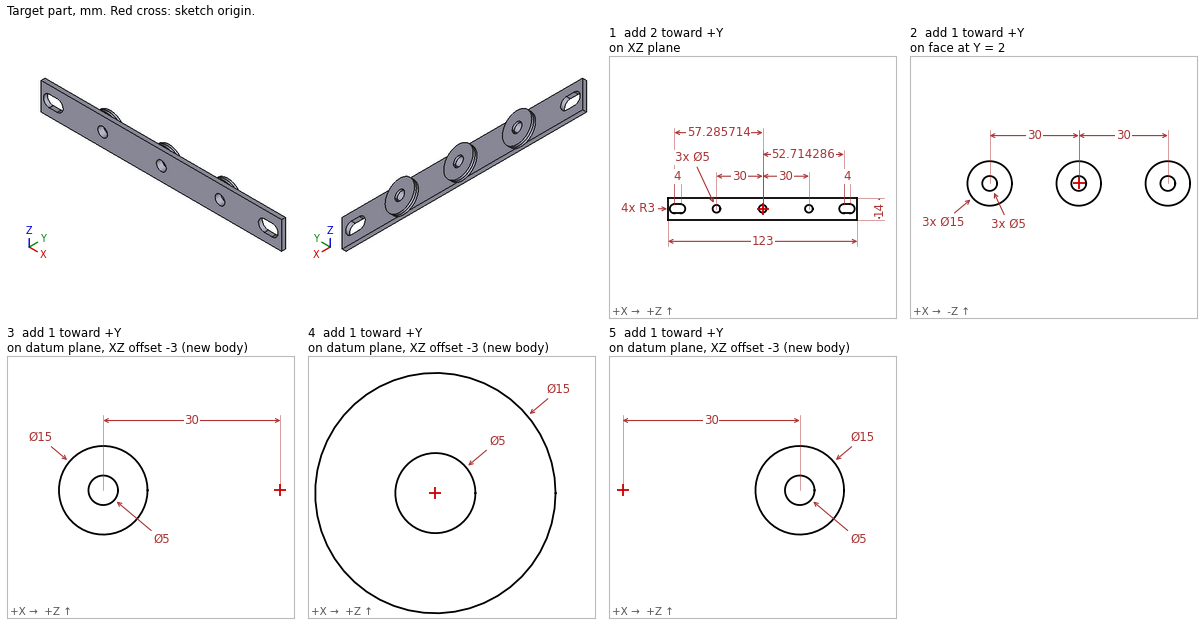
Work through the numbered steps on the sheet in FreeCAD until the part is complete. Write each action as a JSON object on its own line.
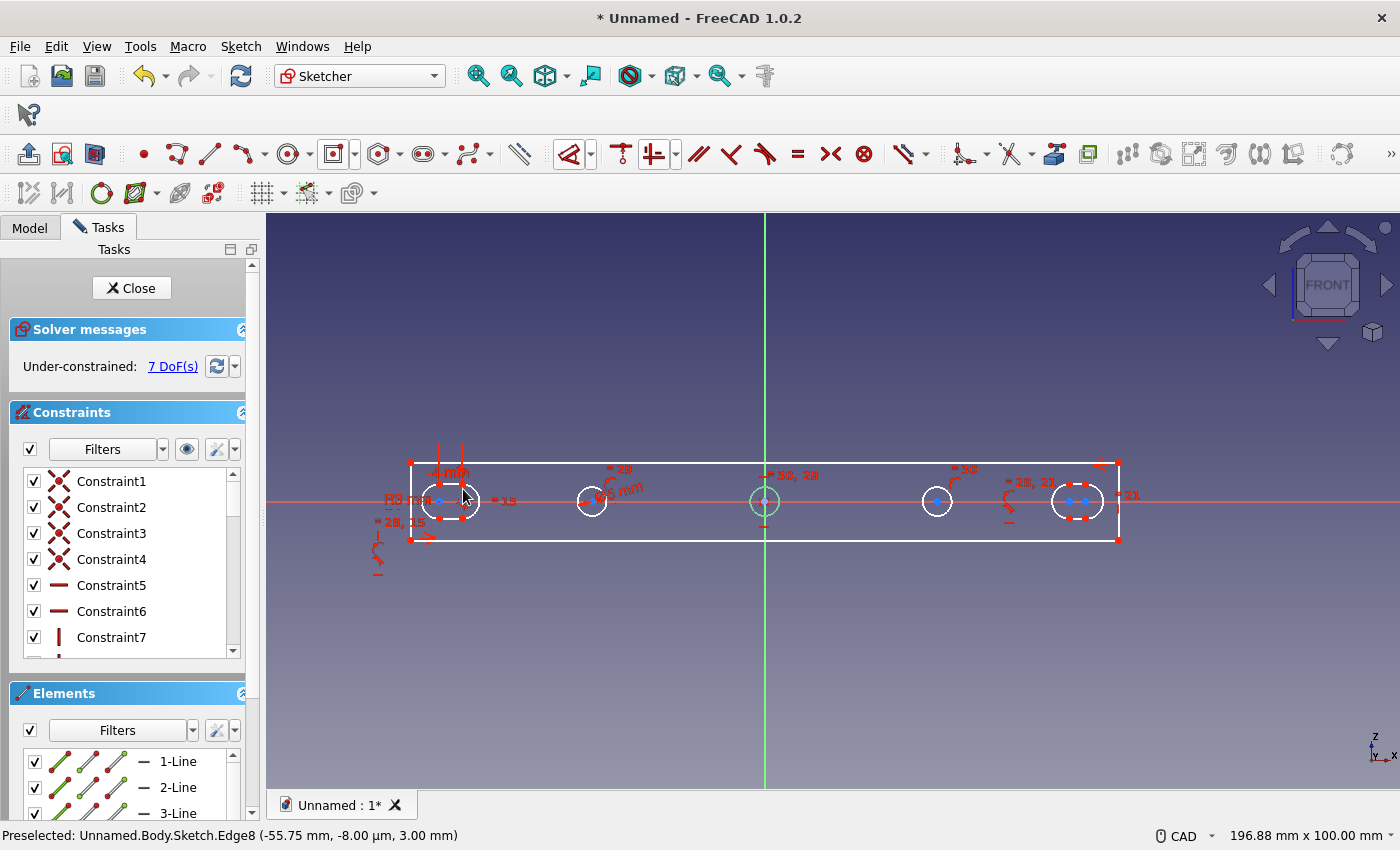
{"action": "scroll", "coordinate": [1074, 484], "scroll_direction": "up", "scroll_amount": 6}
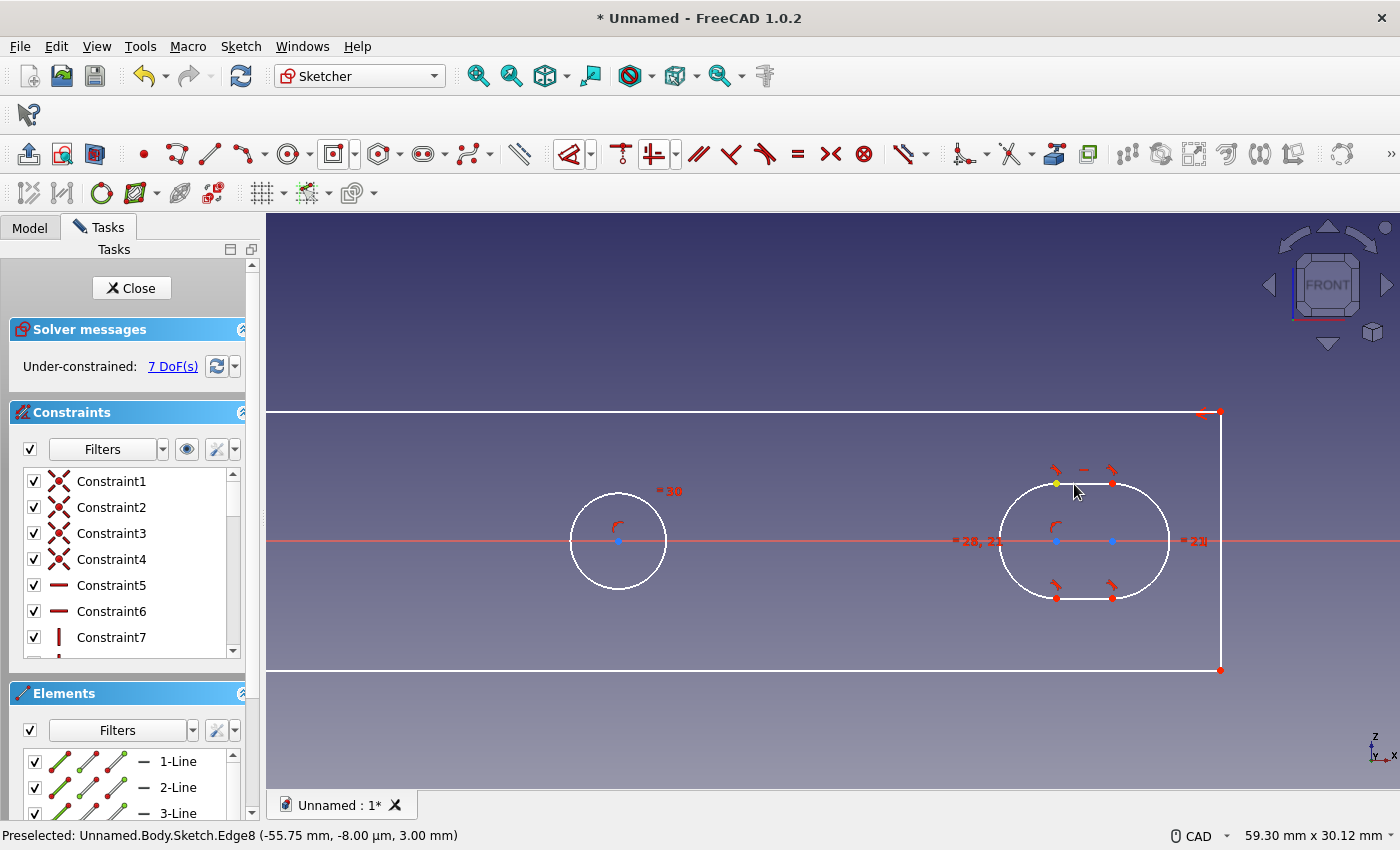
{"action": "left_click", "coordinate": [1073, 484]}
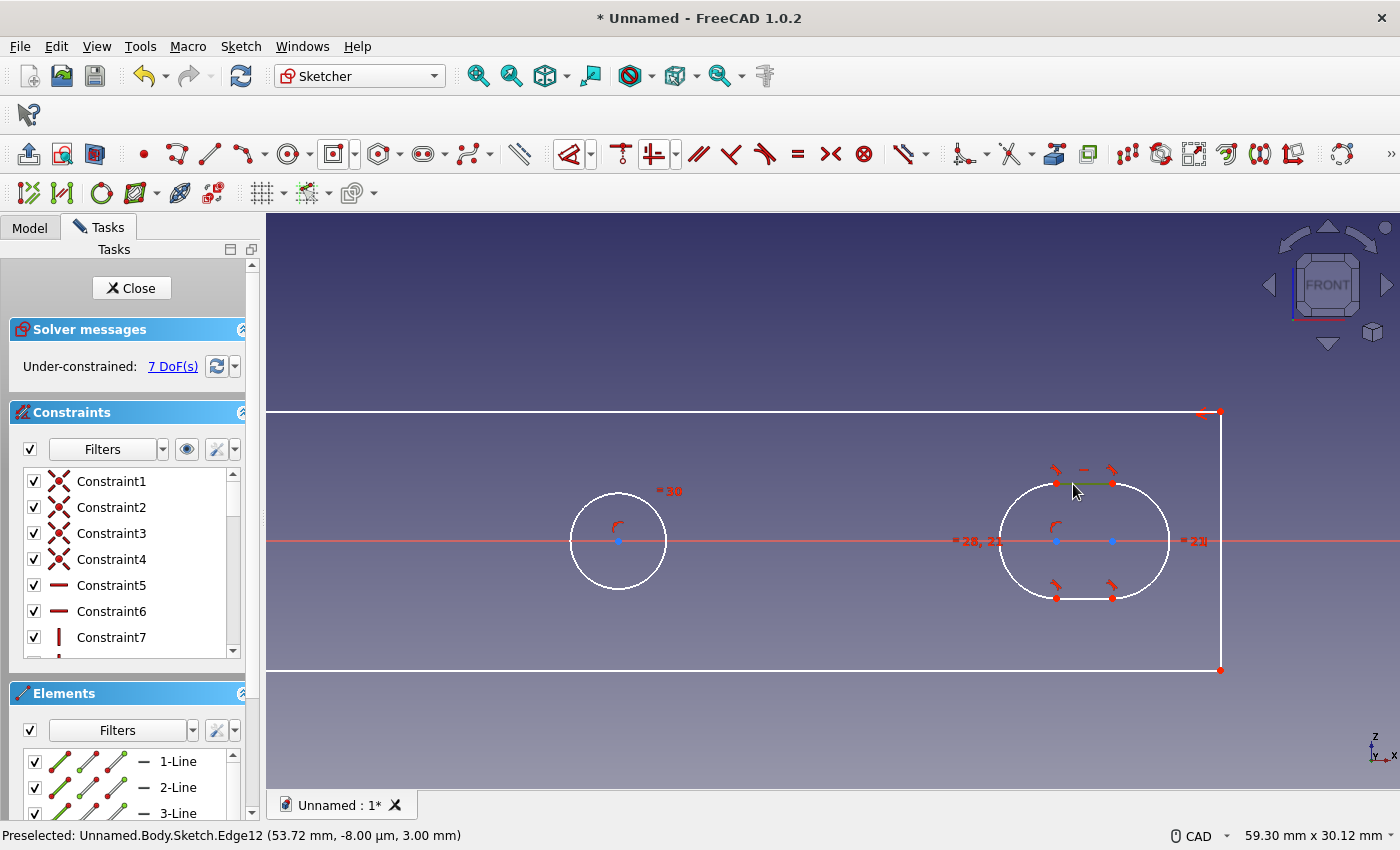
{"action": "left_click", "coordinate": [590, 154]}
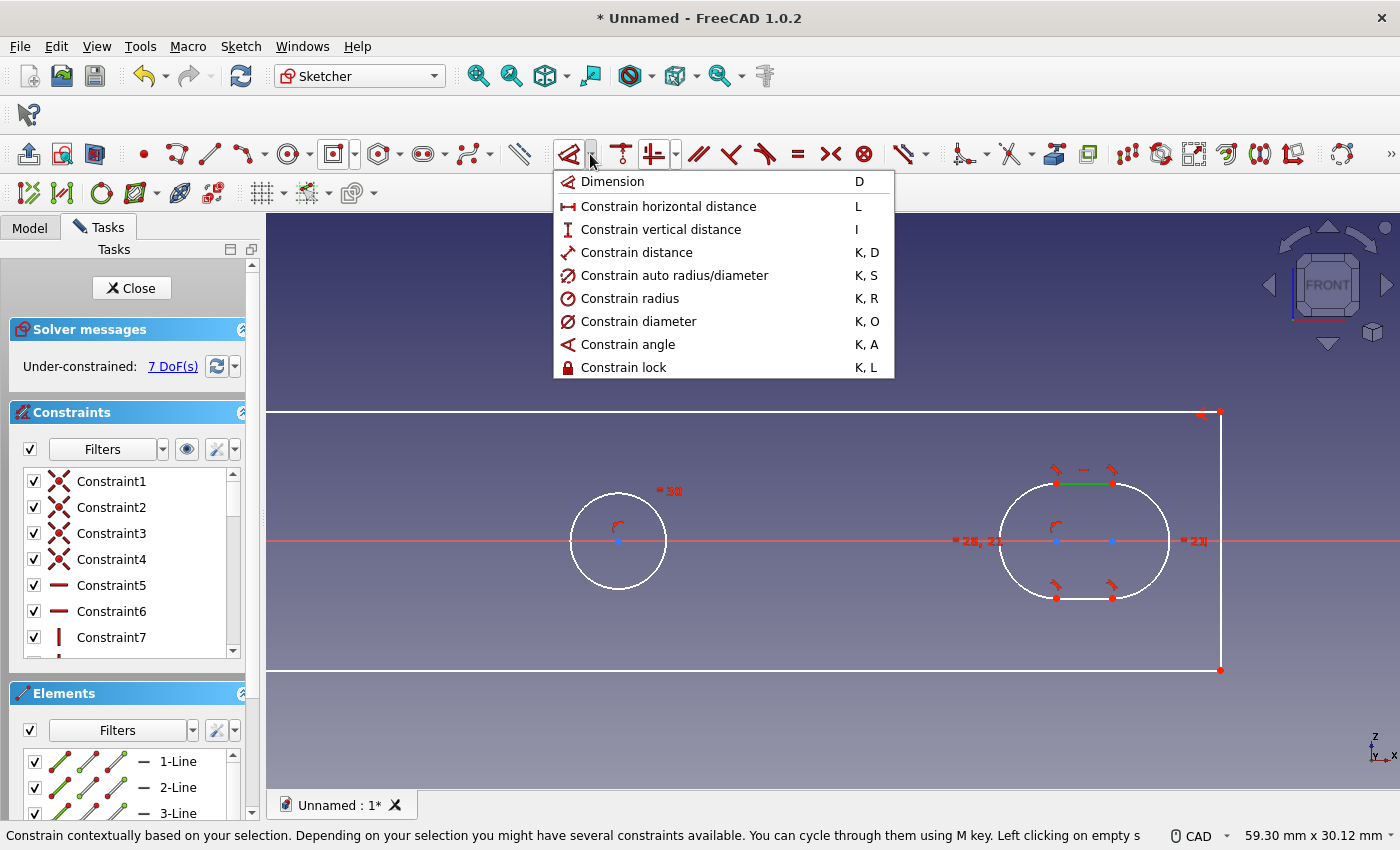
{"action": "left_click", "coordinate": [724, 206]}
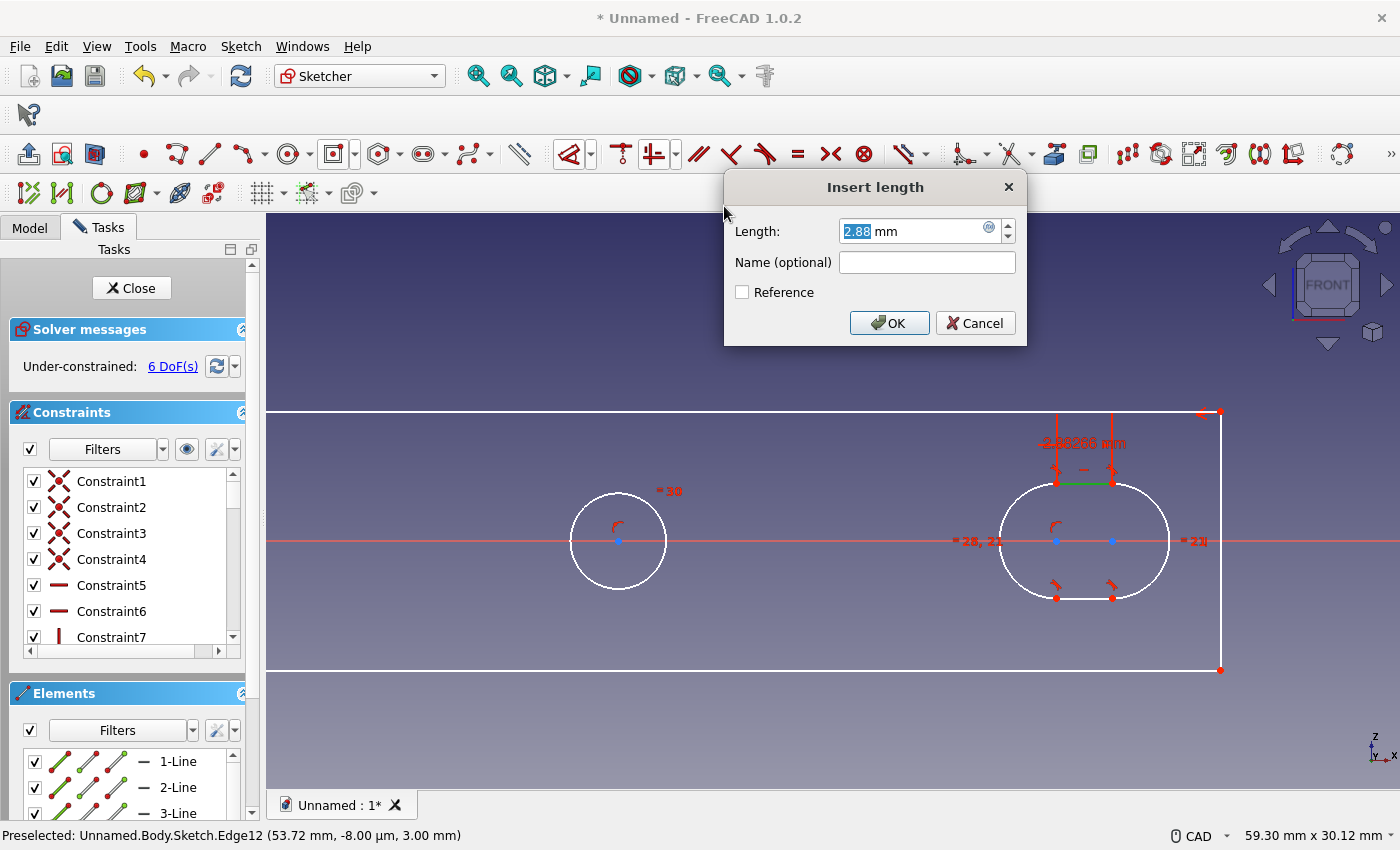
{"action": "type", "text": "4"}
{"action": "key", "text": "Return"}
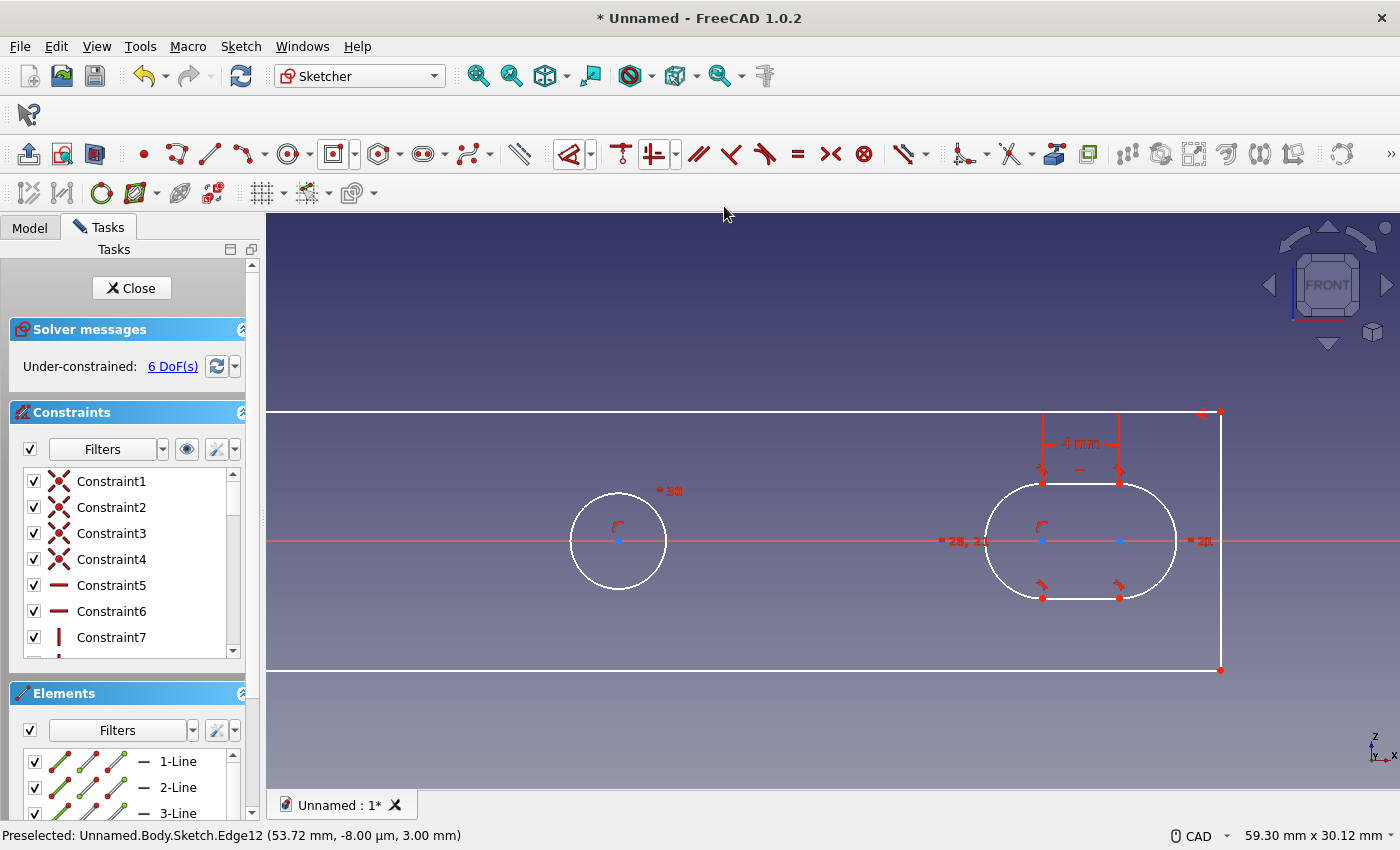
{"action": "left_click", "coordinate": [1221, 593]}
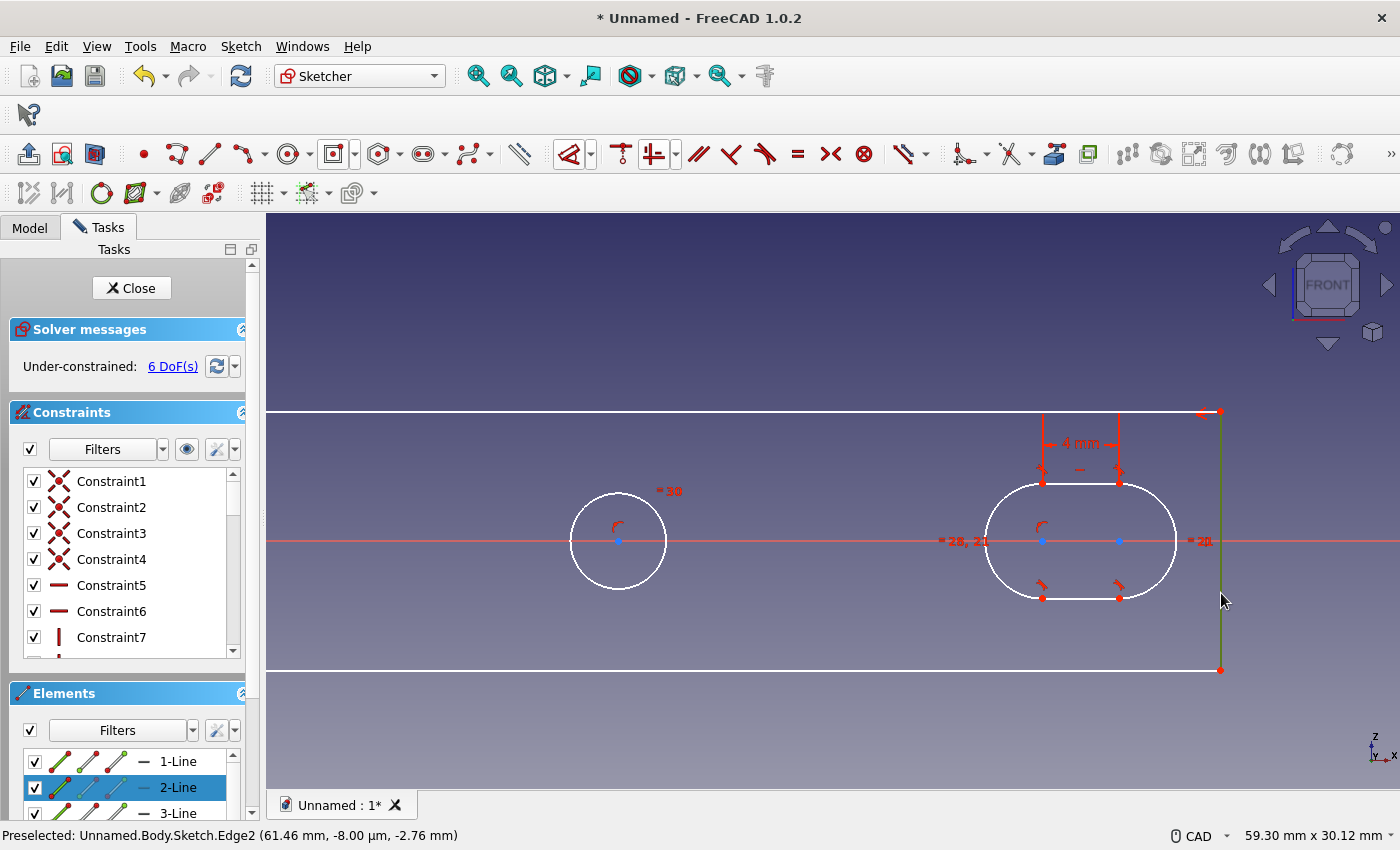
{"action": "left_click", "coordinate": [590, 154]}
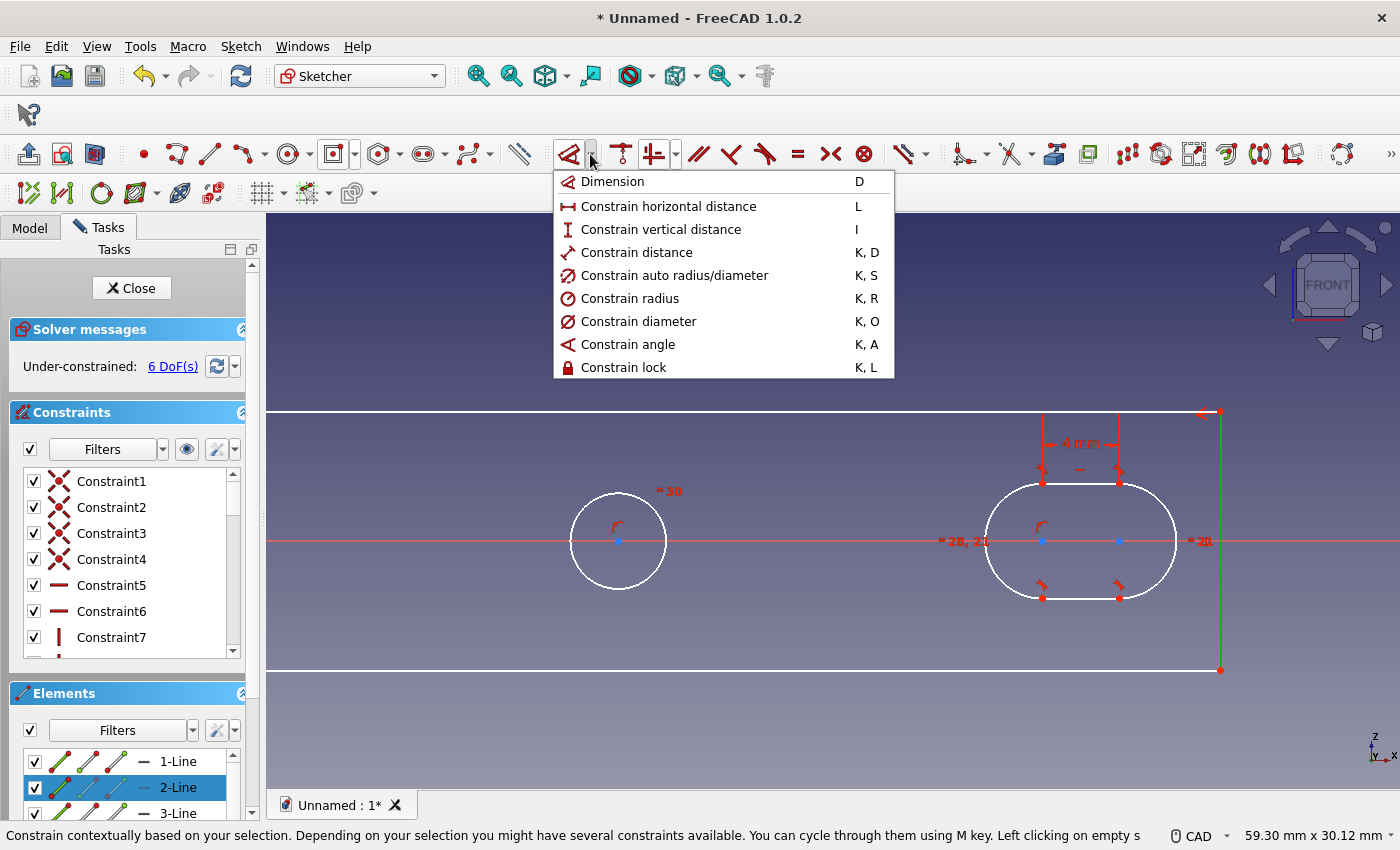
{"action": "left_click", "coordinate": [724, 230]}